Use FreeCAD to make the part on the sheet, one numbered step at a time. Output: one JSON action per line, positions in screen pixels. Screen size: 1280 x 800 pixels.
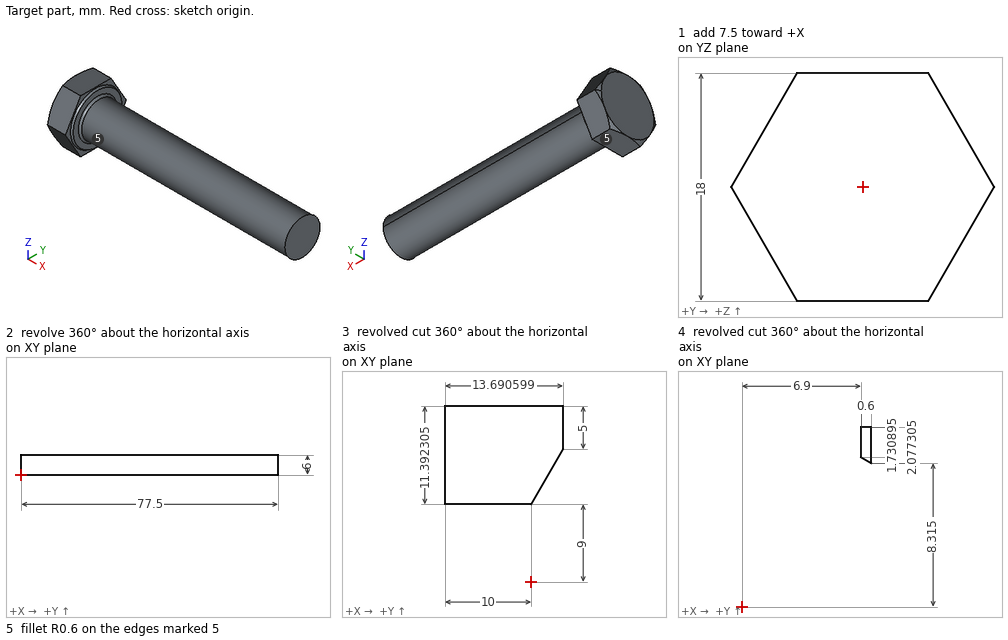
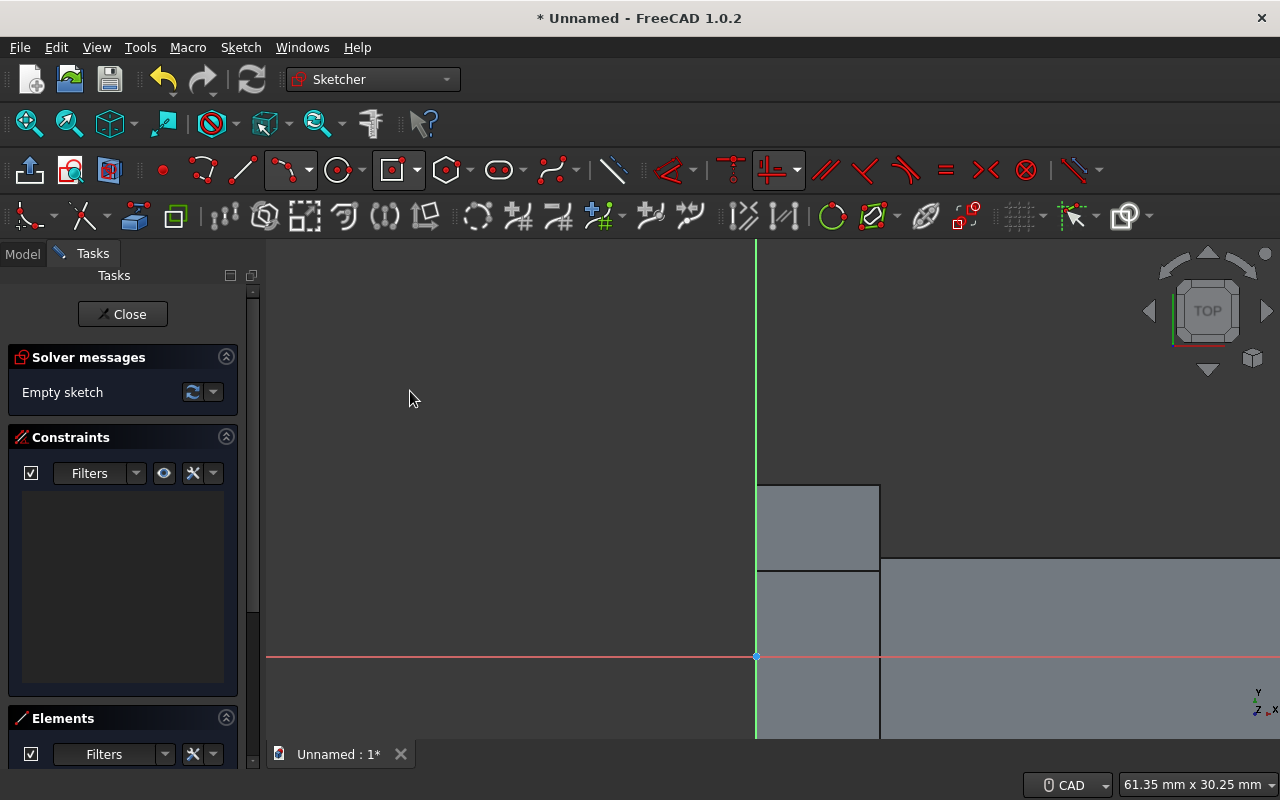
{"action": "left_click", "coordinate": [204, 170]}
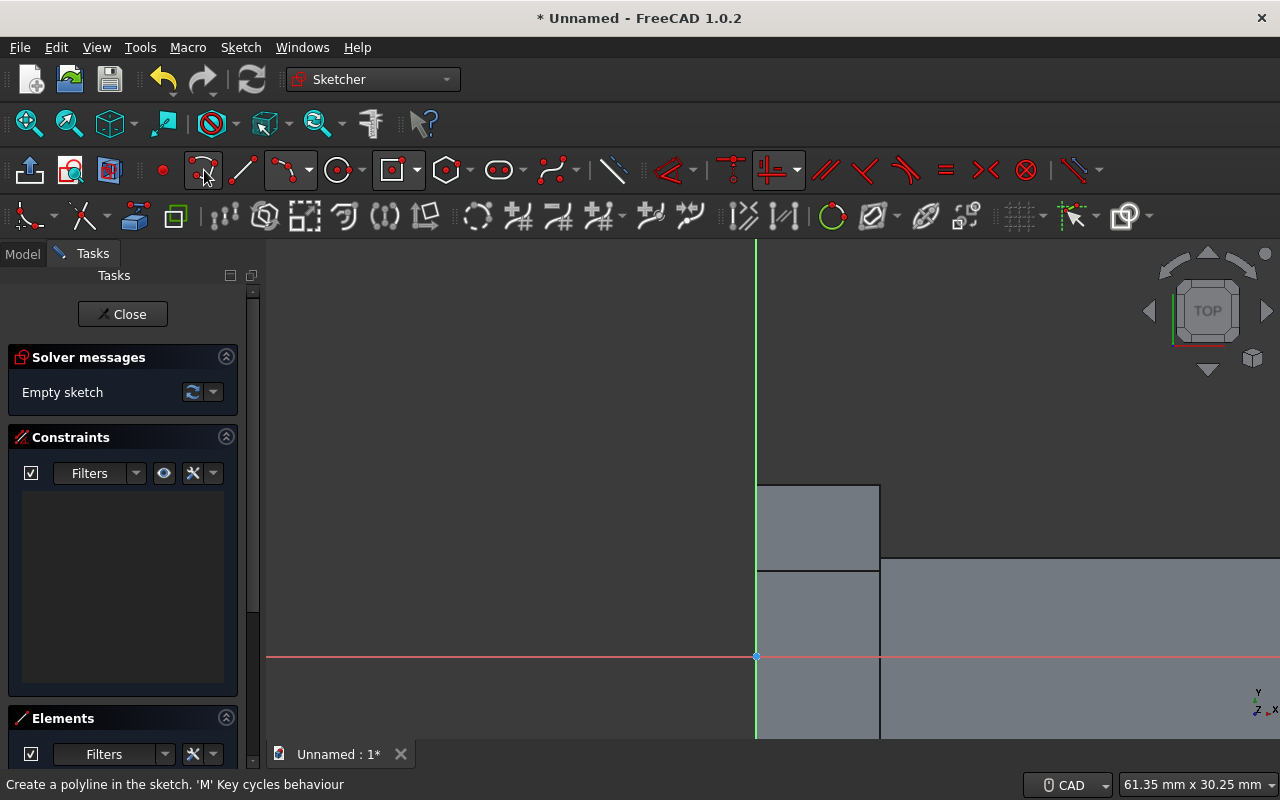
{"action": "left_click", "coordinate": [756, 508]}
{"action": "left_click", "coordinate": [817, 402]}
{"action": "left_click", "coordinate": [817, 320]}
{"action": "left_click", "coordinate": [591, 320]}
{"action": "left_click", "coordinate": [591, 508]}
{"action": "left_click", "coordinate": [756, 509]}
{"action": "key", "text": "Escape"}
{"action": "key", "text": "Escape"}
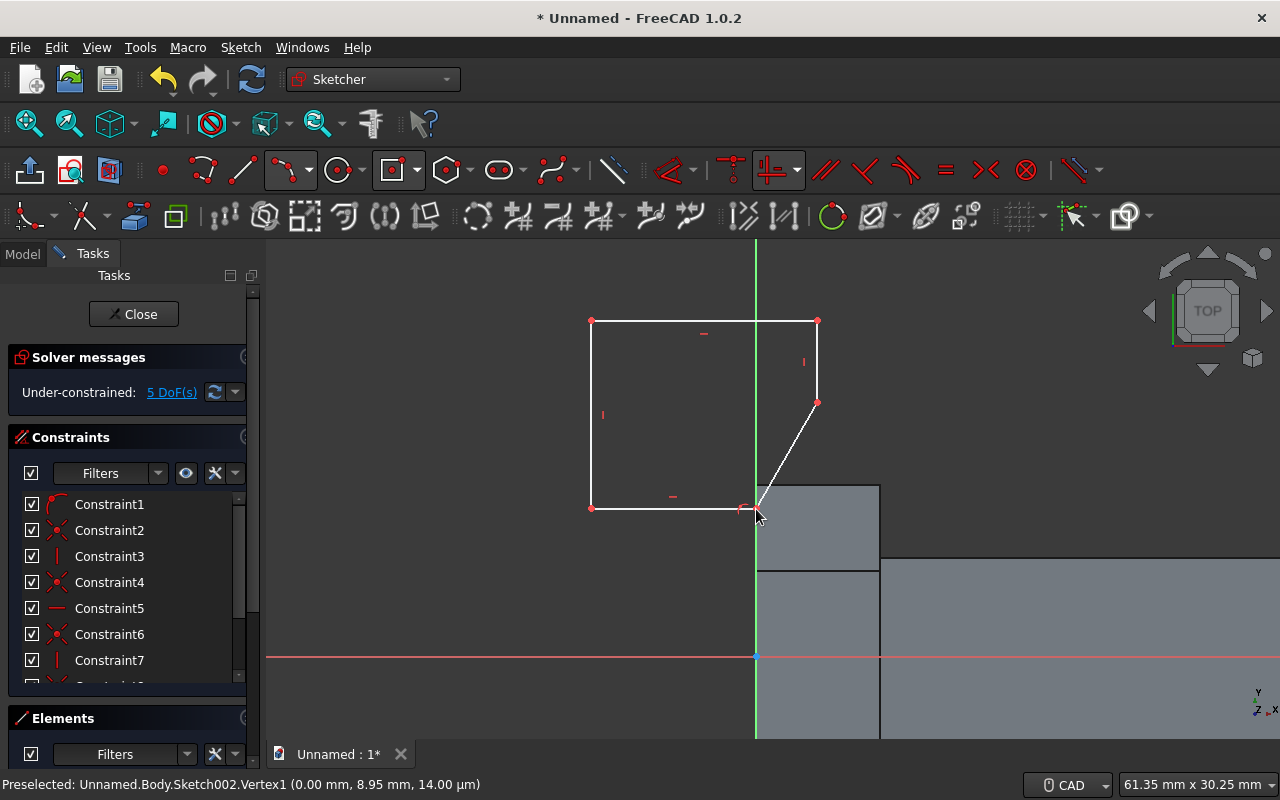
{"action": "left_click", "coordinate": [668, 170]}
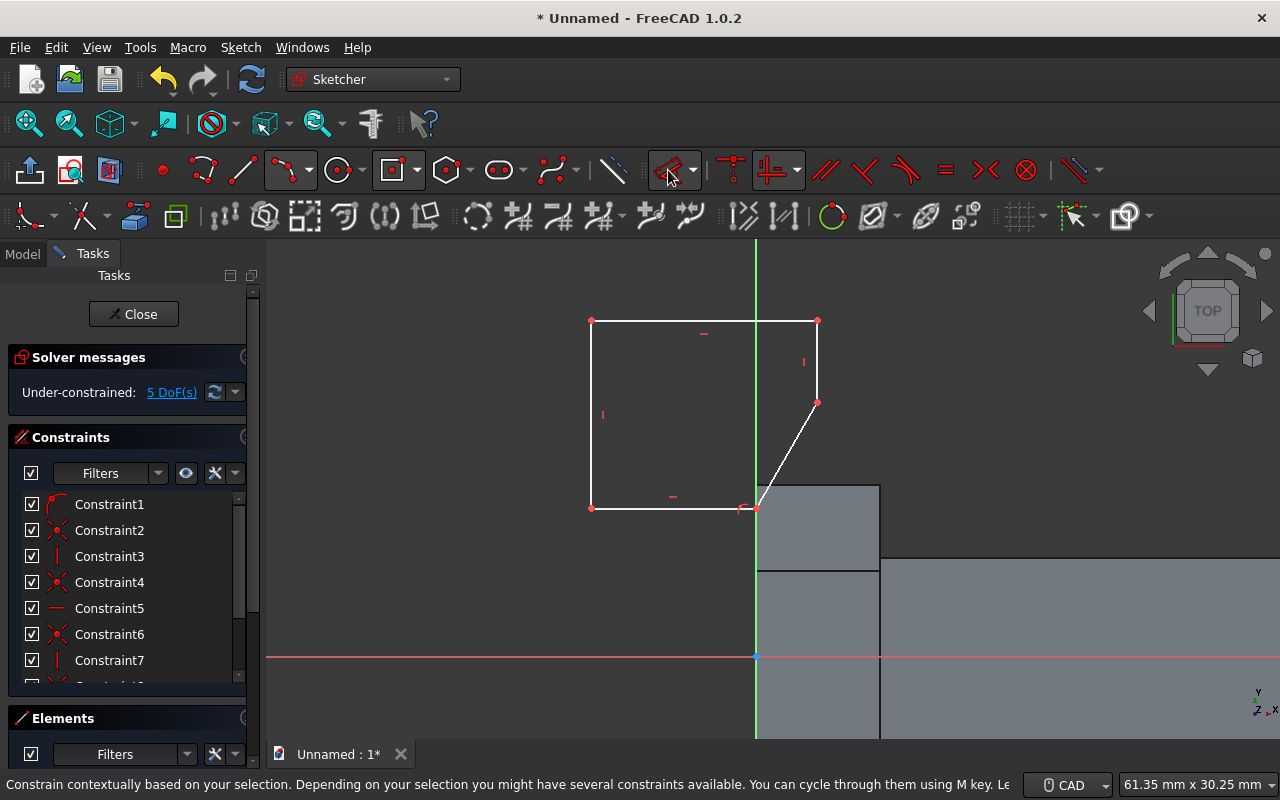
{"action": "left_click", "coordinate": [817, 378]}
{"action": "left_click", "coordinate": [851, 362]}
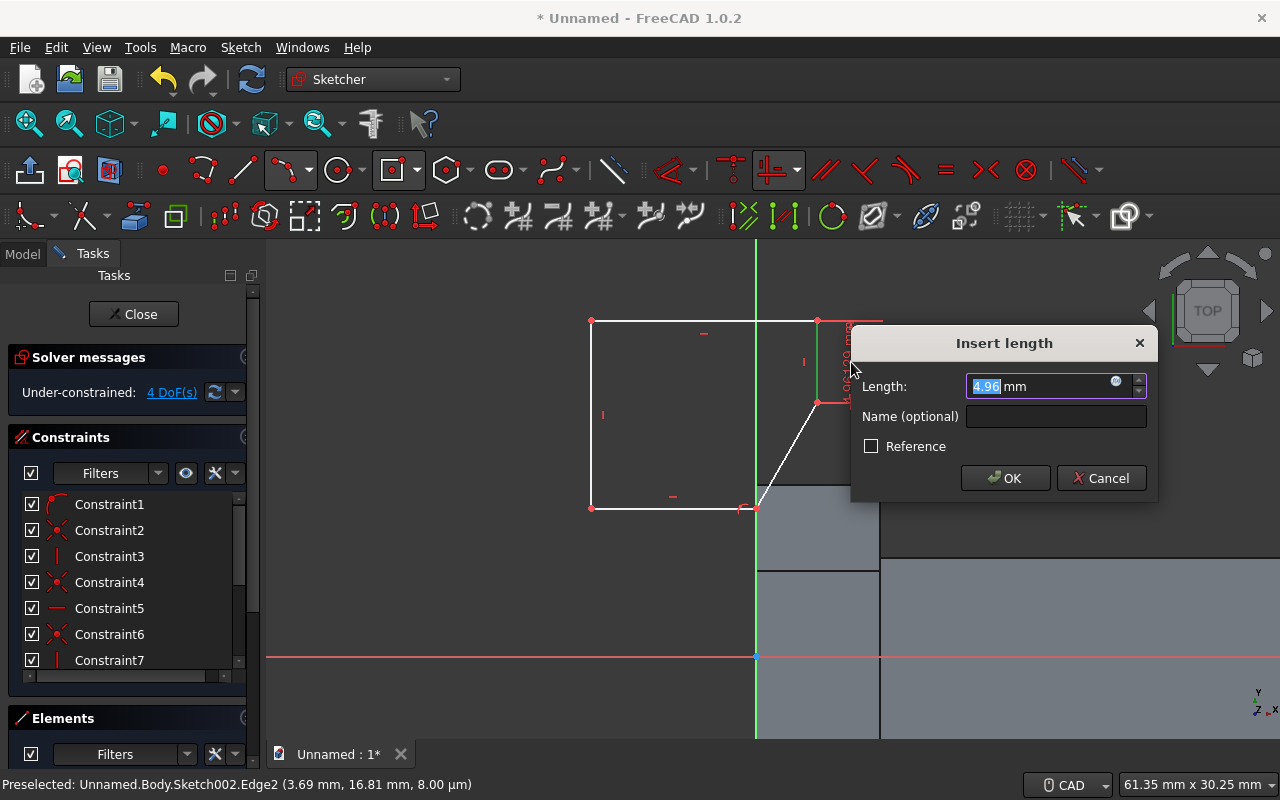
{"action": "type", "text": "5"}
{"action": "key", "text": "Return"}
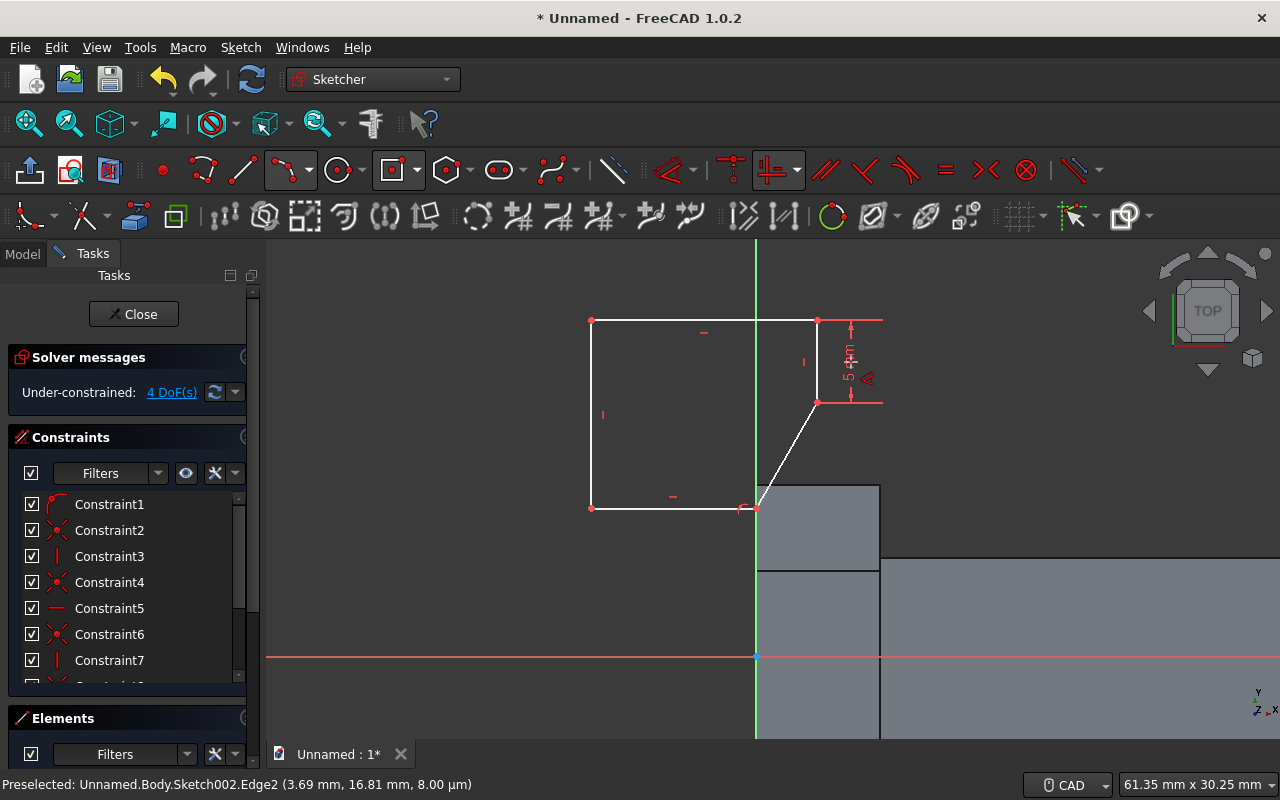
{"action": "left_click", "coordinate": [641, 509]}
{"action": "left_click", "coordinate": [674, 543]}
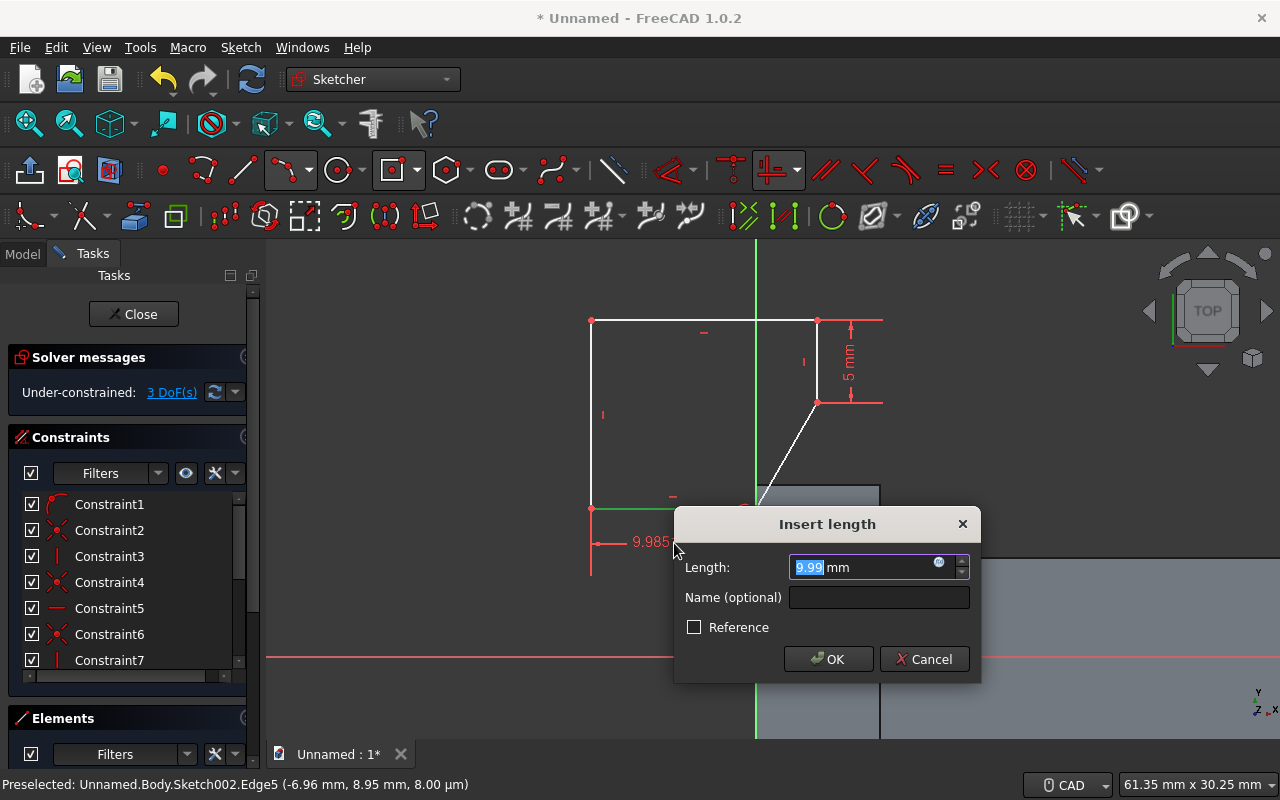
{"action": "type", "text": "10"}
{"action": "key", "text": "Return"}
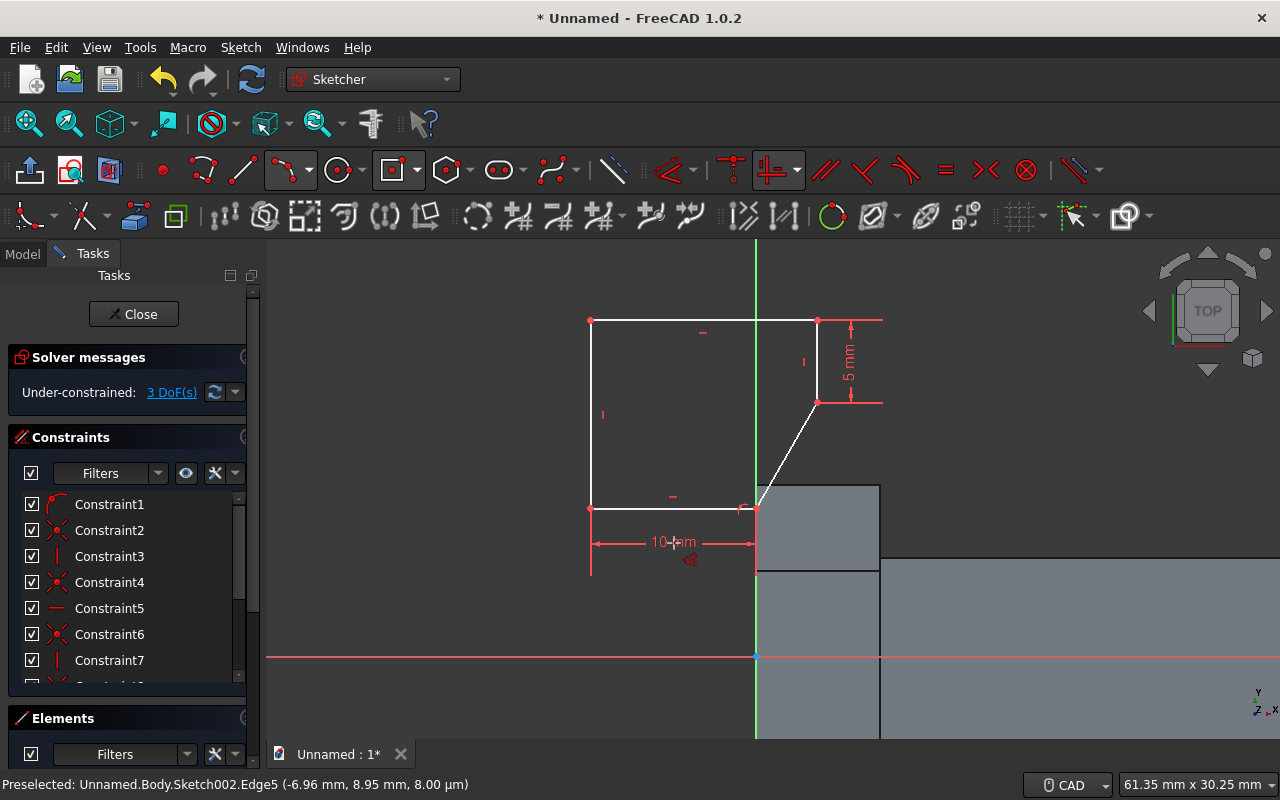
{"action": "left_click", "coordinate": [756, 509]}
{"action": "left_click", "coordinate": [790, 583]}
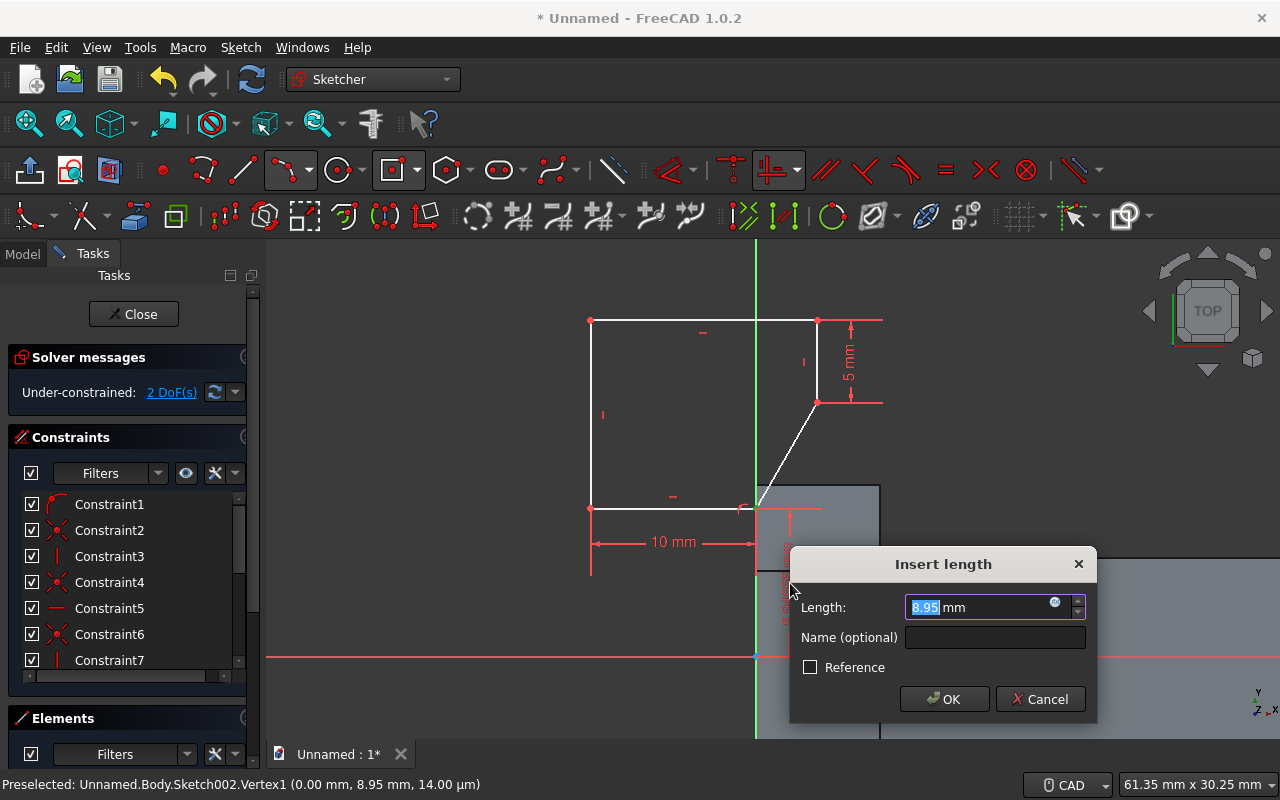
{"action": "type", "text": "9"}
{"action": "key", "text": "Return"}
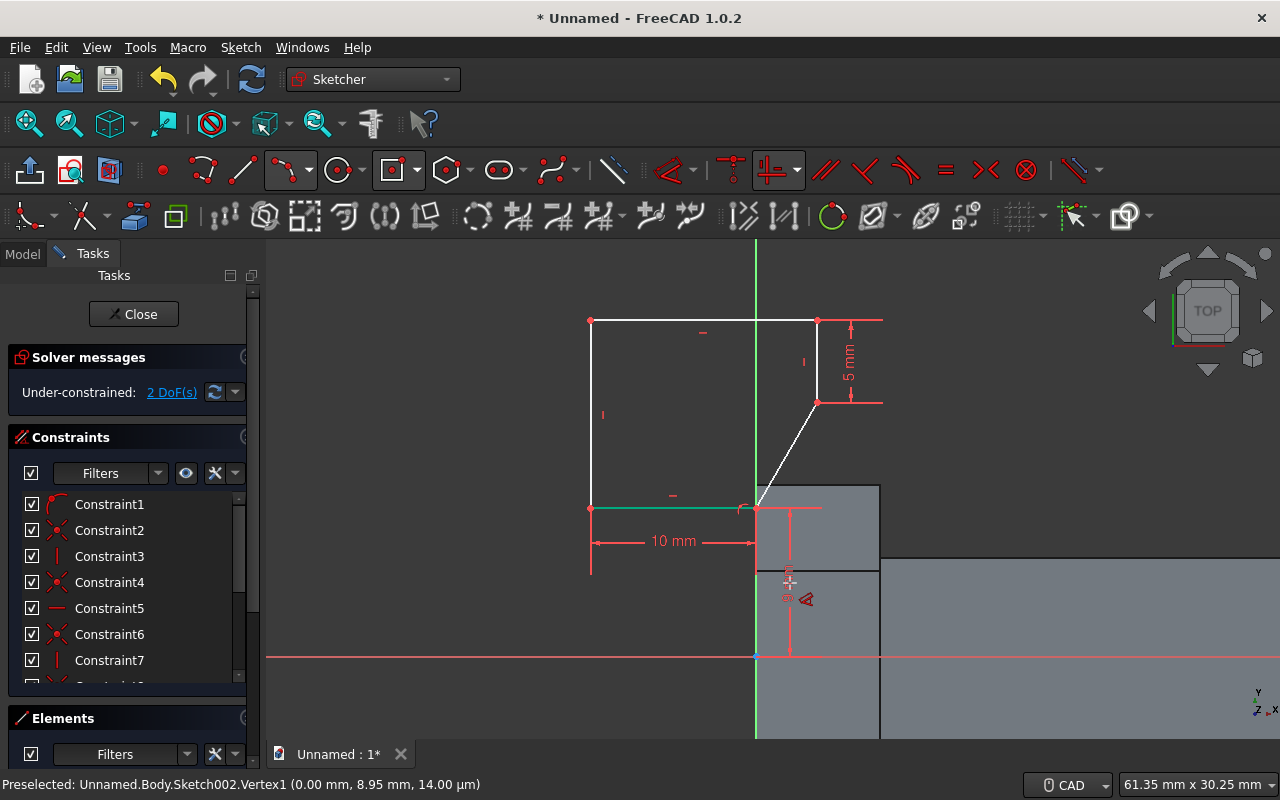
{"action": "left_click", "coordinate": [659, 320]}
{"action": "left_click", "coordinate": [704, 286]}